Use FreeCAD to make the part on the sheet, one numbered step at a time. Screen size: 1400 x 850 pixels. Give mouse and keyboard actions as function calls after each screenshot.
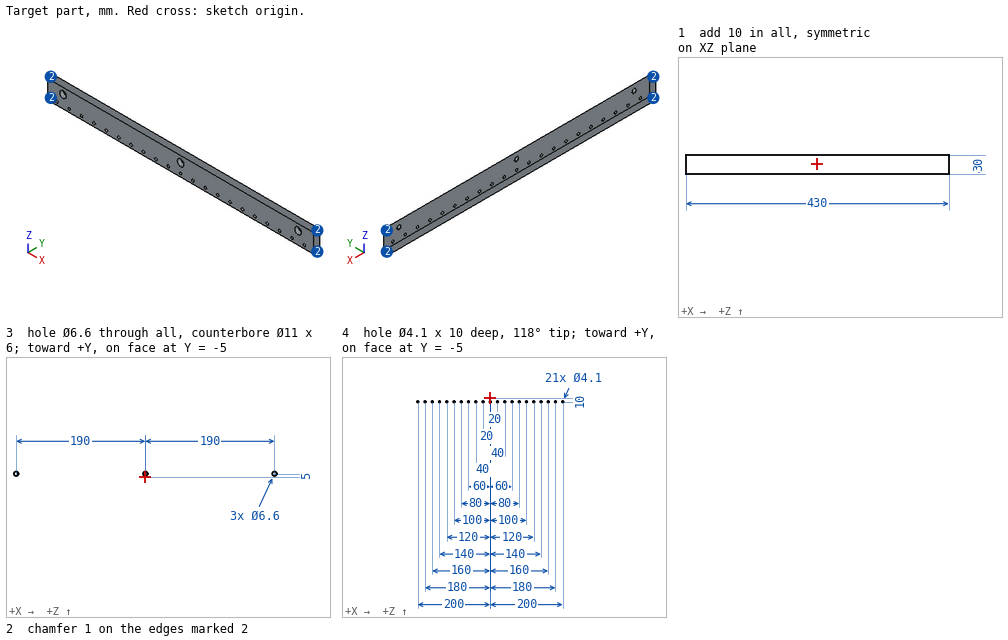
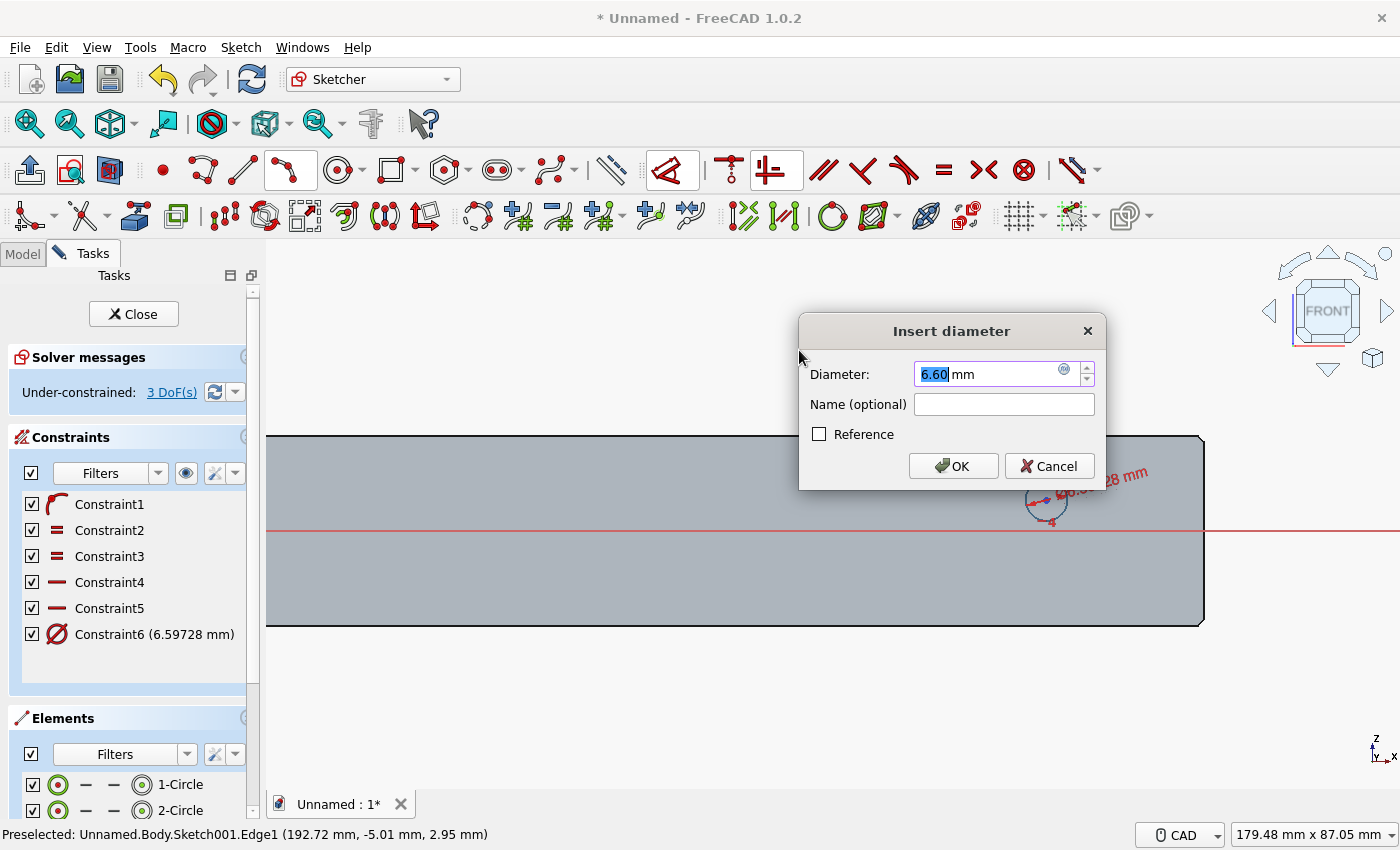
text(6.6)
key(Return)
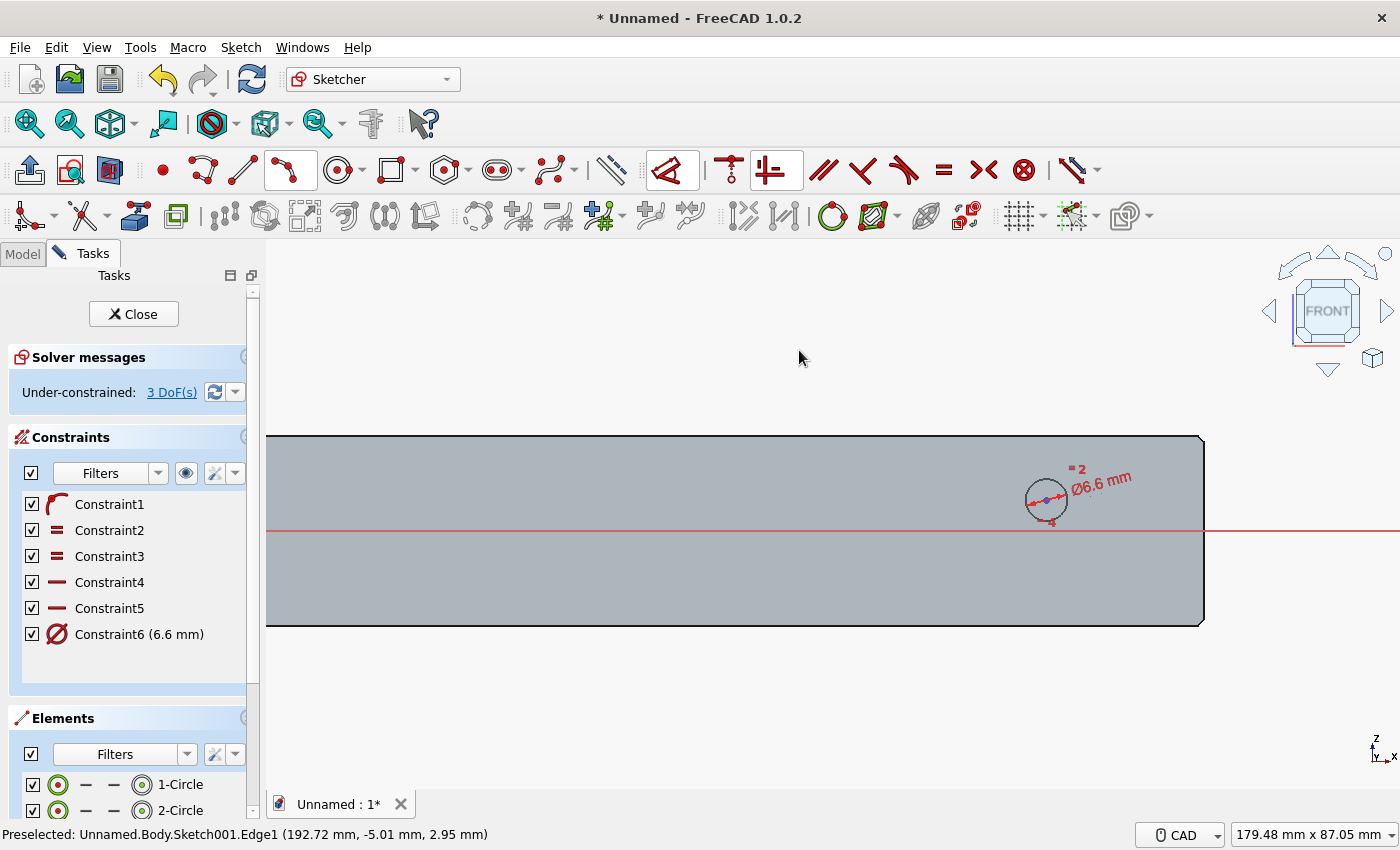
scroll(1047, 500, up, 2)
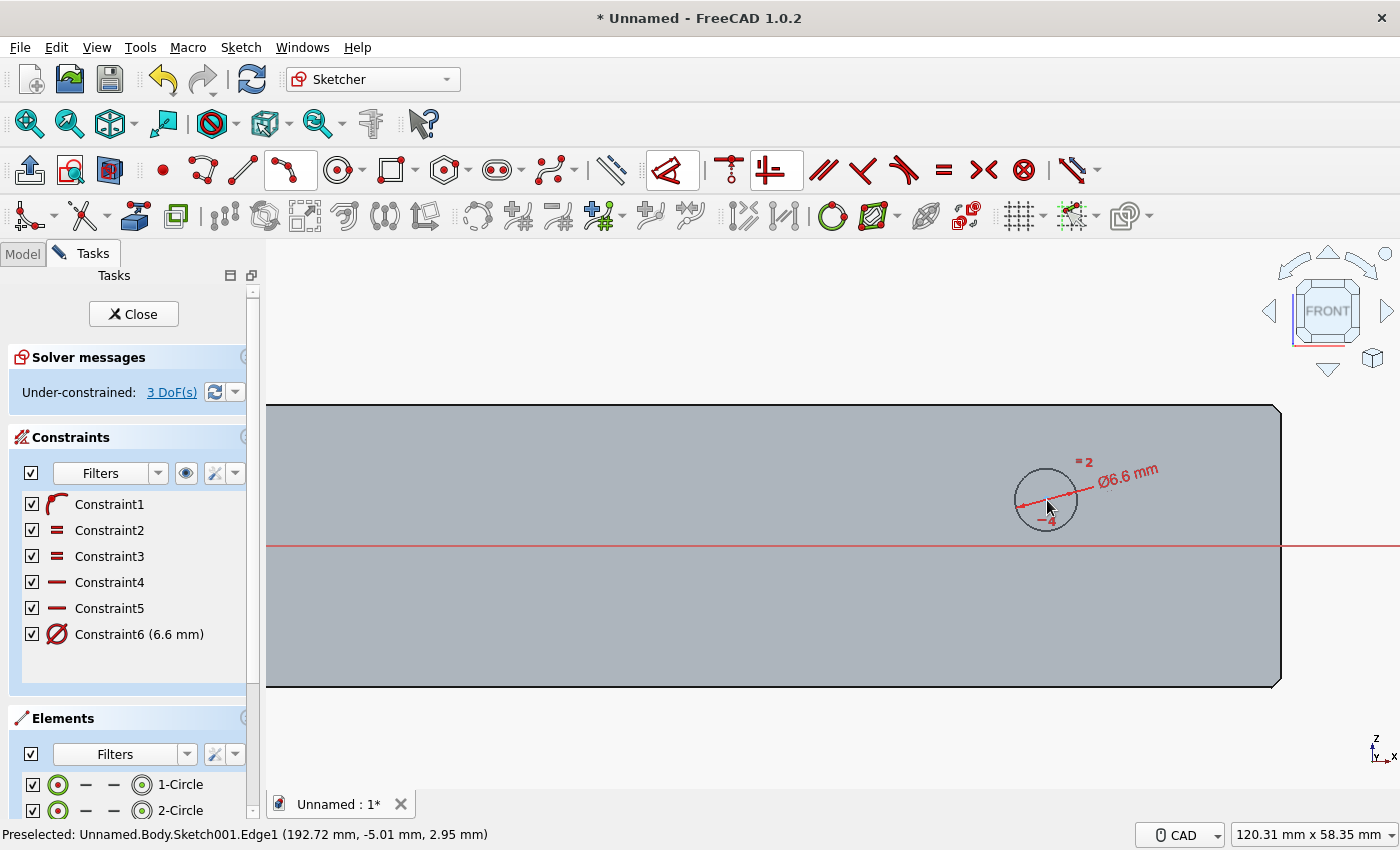
click(1046, 500)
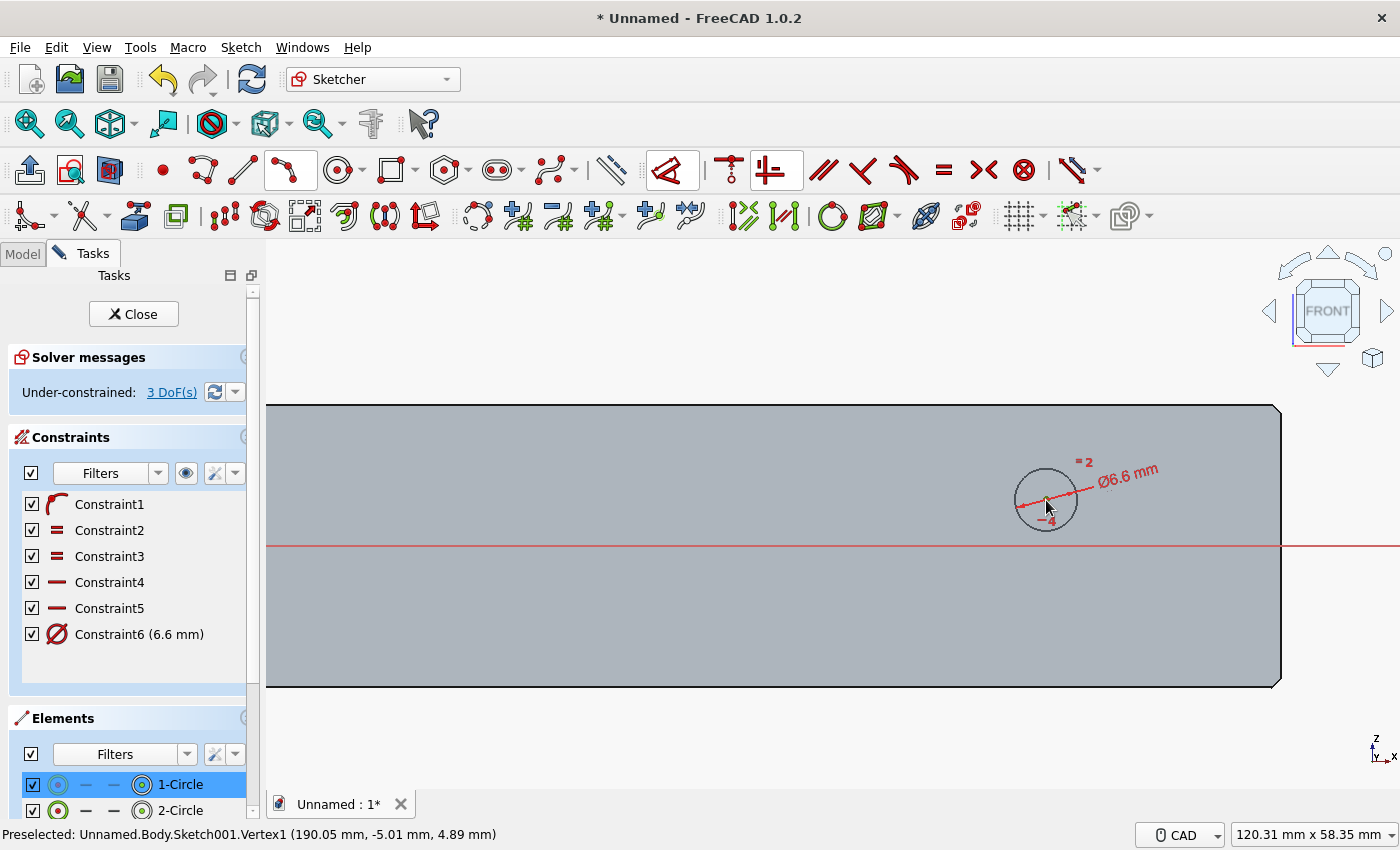
key(i)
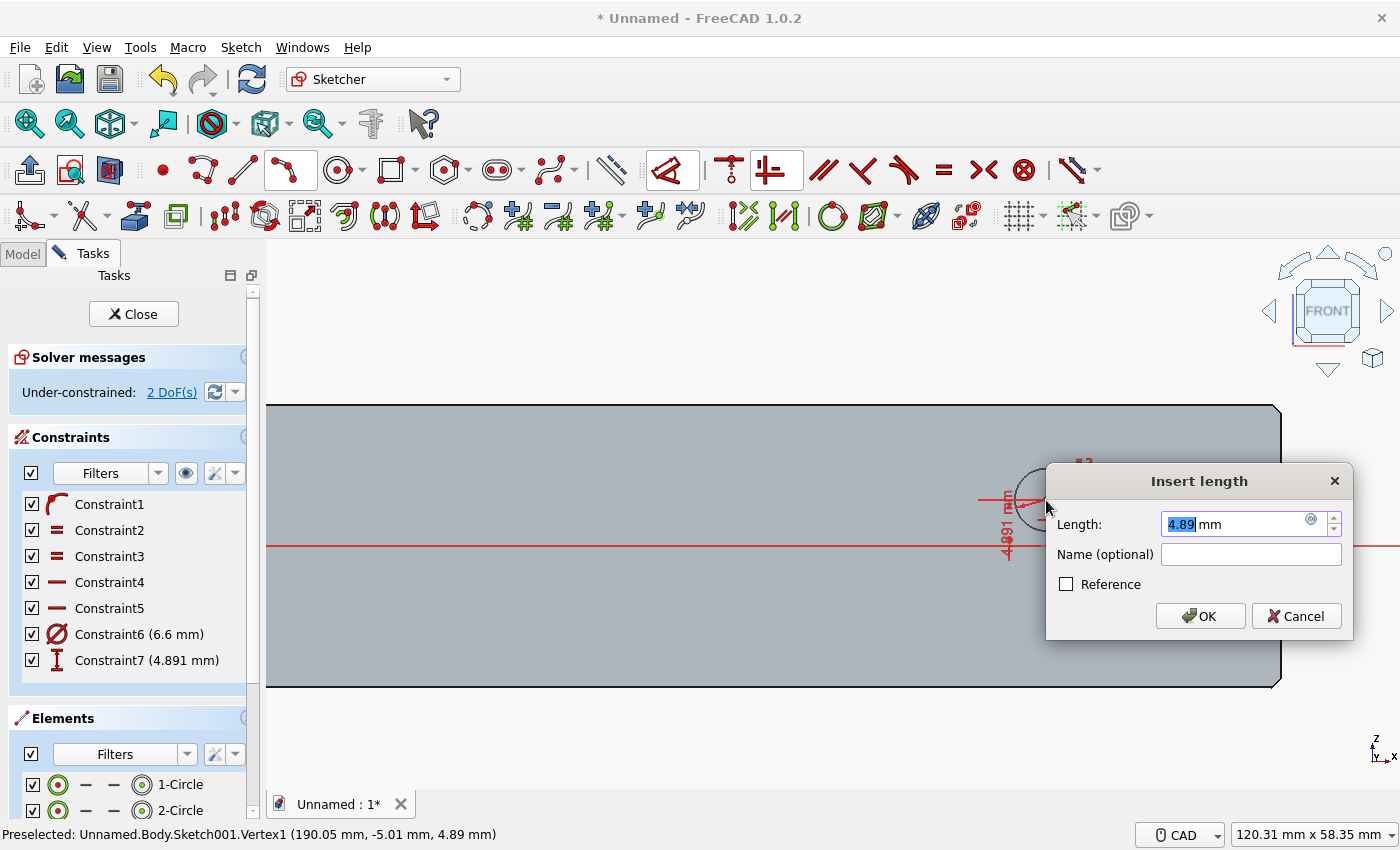
text(5)
key(Return)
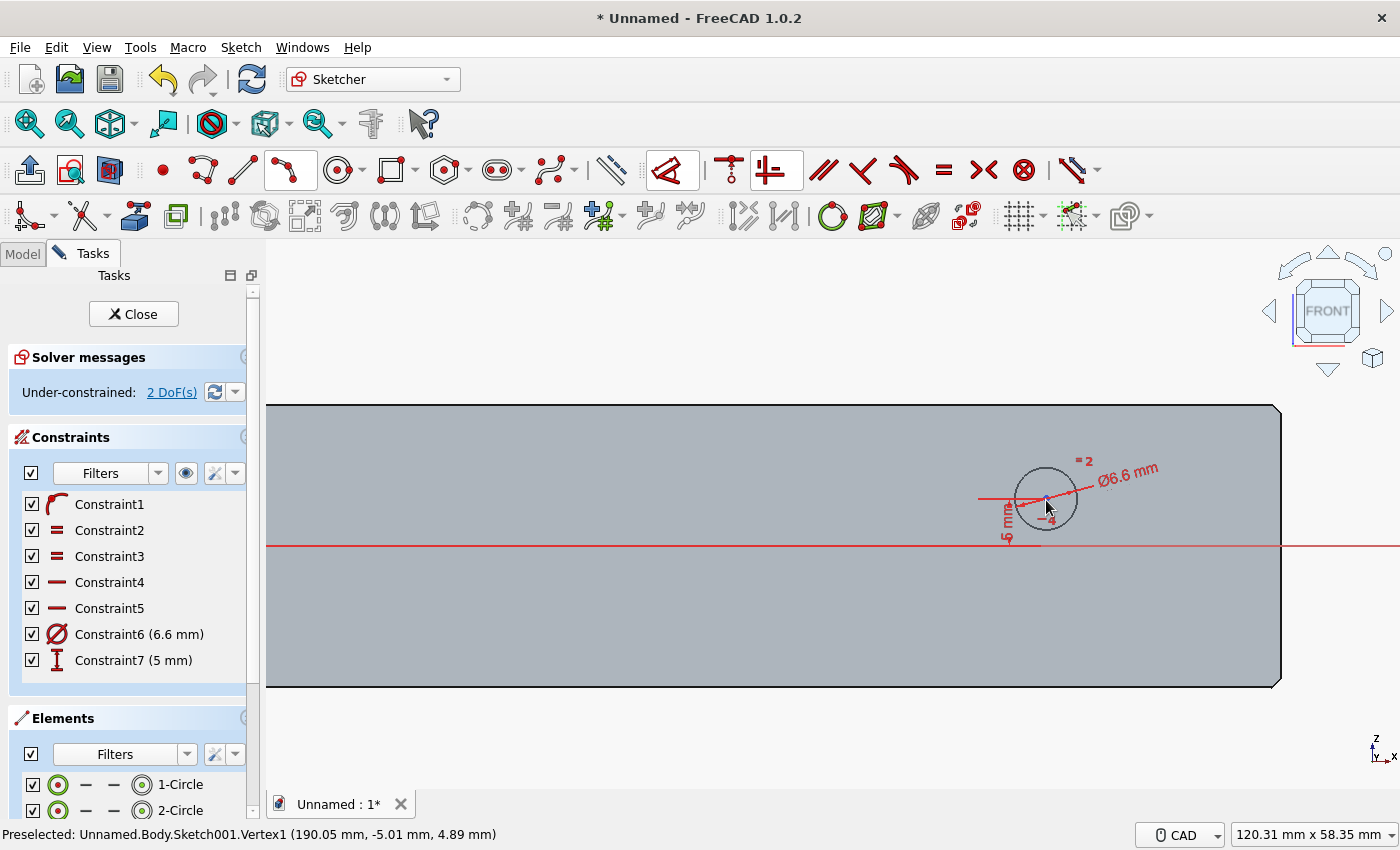
scroll(1063, 515, down, 9)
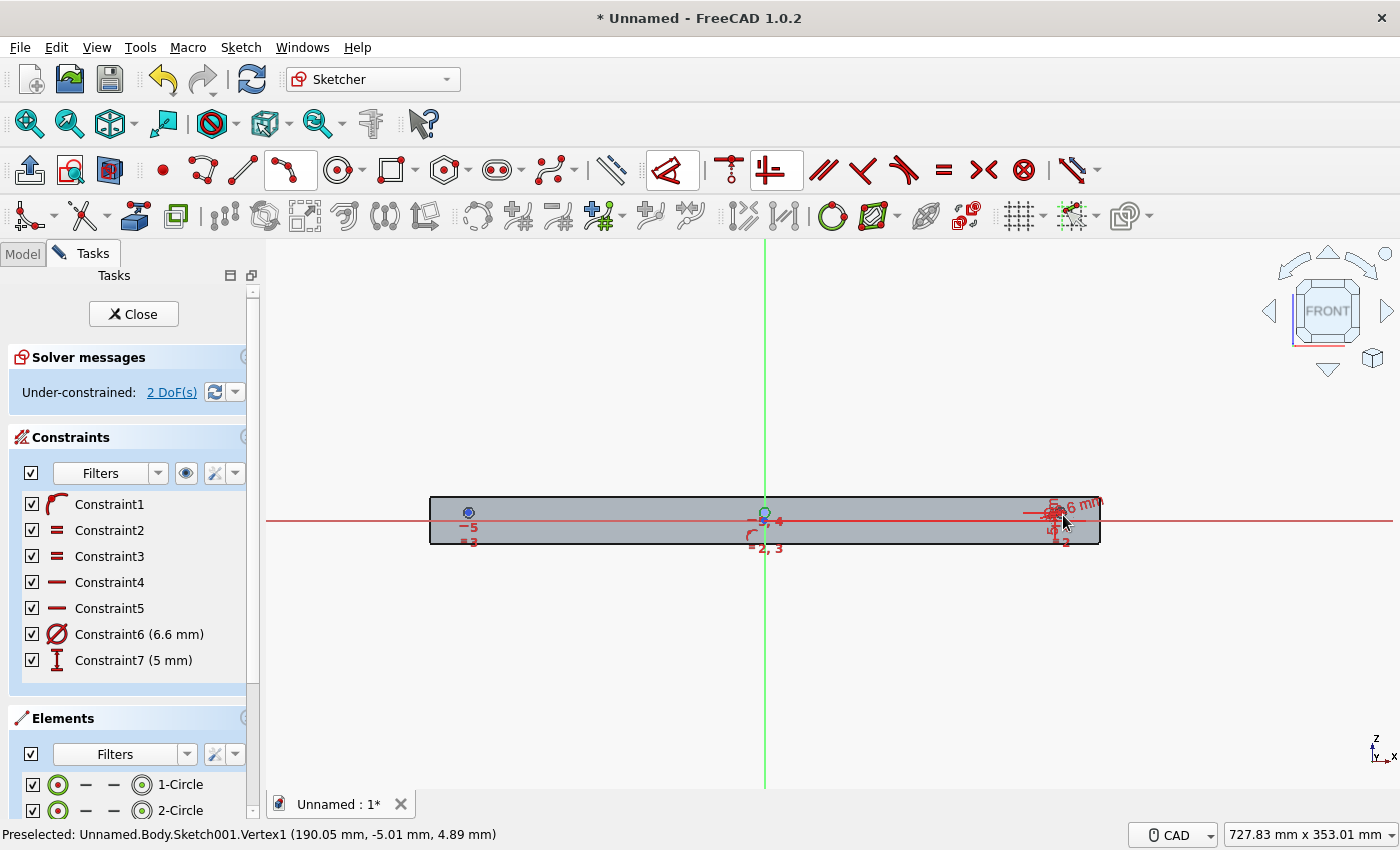
click(1061, 513)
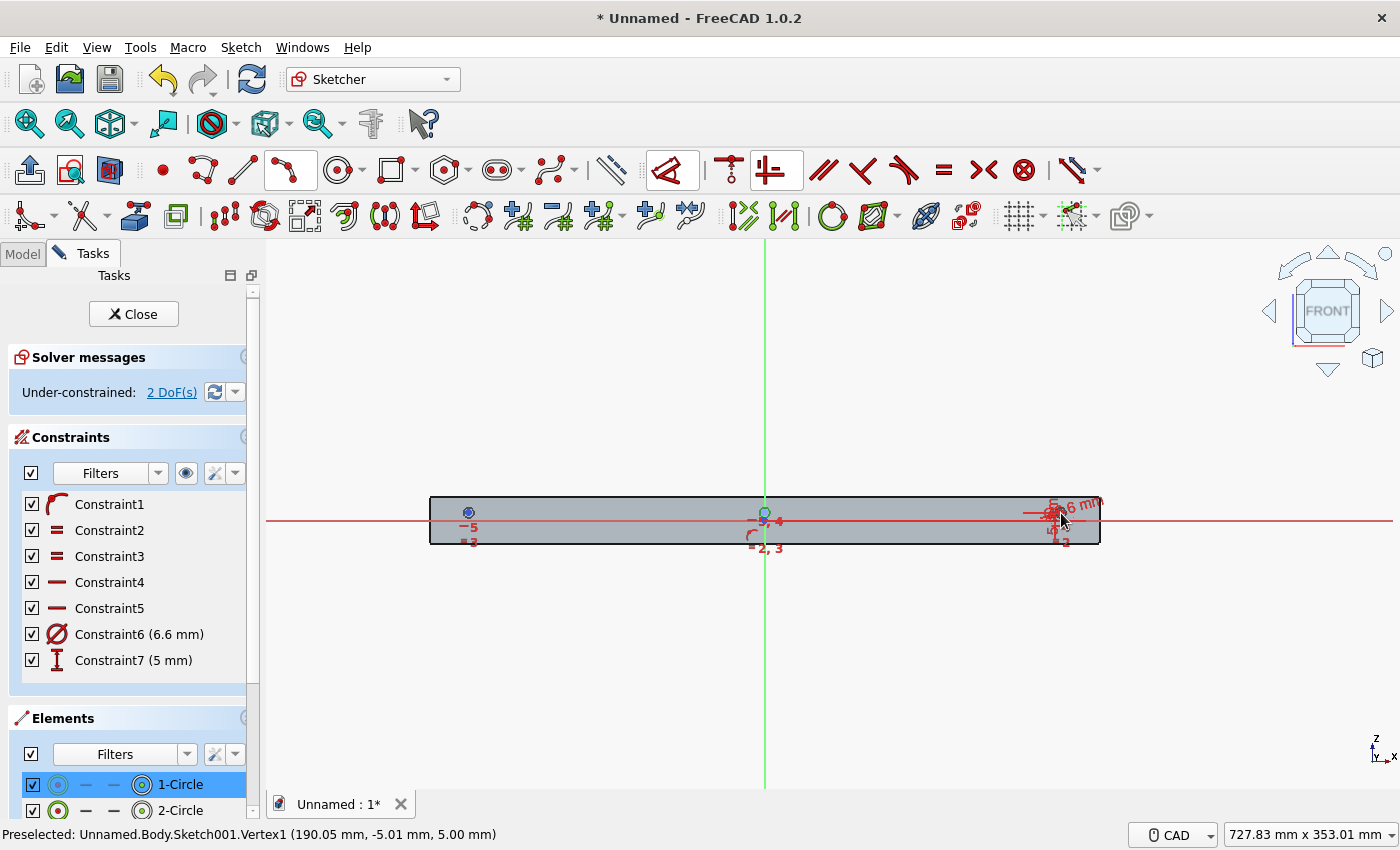
key(l)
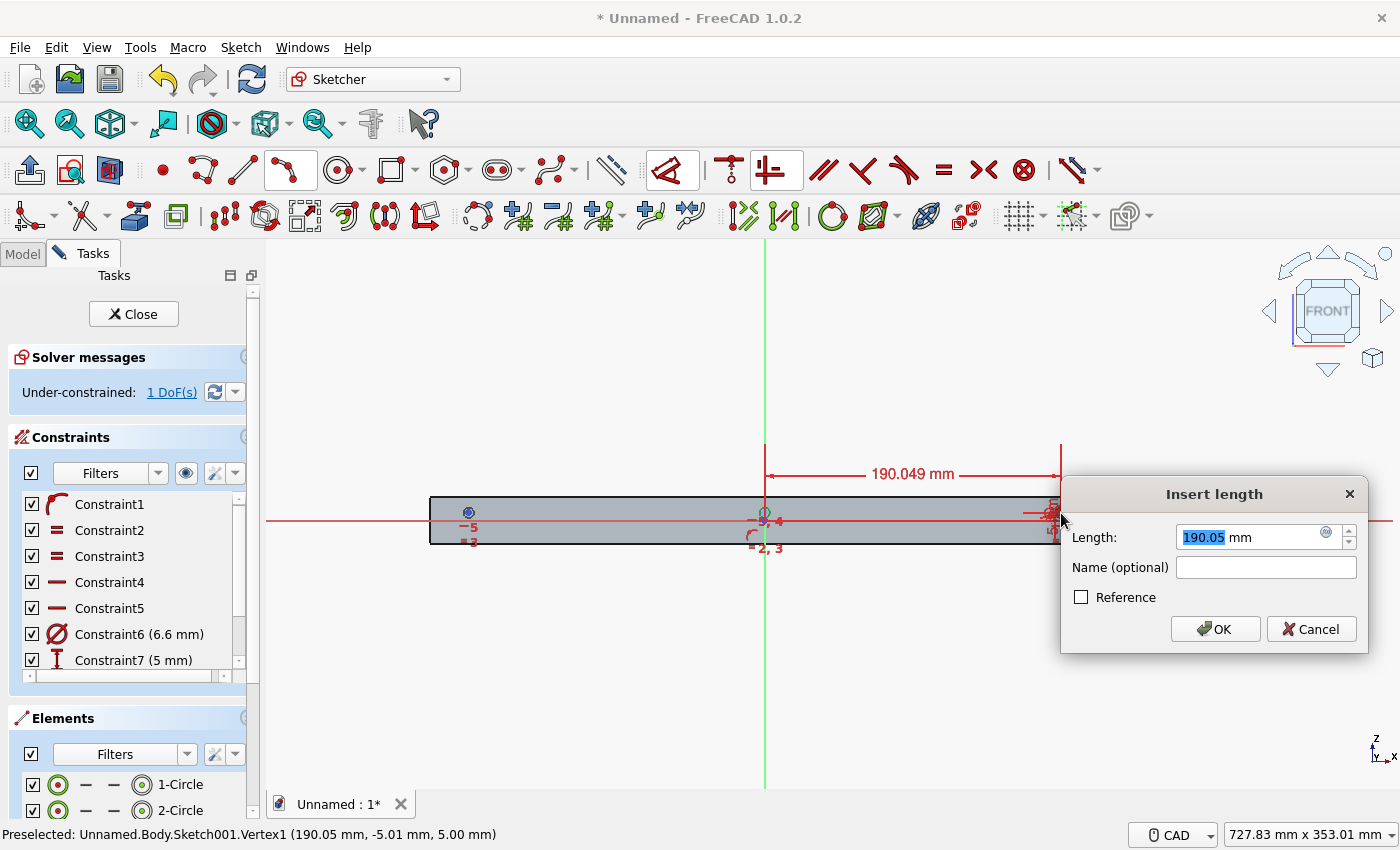
text(190)
key(Return)